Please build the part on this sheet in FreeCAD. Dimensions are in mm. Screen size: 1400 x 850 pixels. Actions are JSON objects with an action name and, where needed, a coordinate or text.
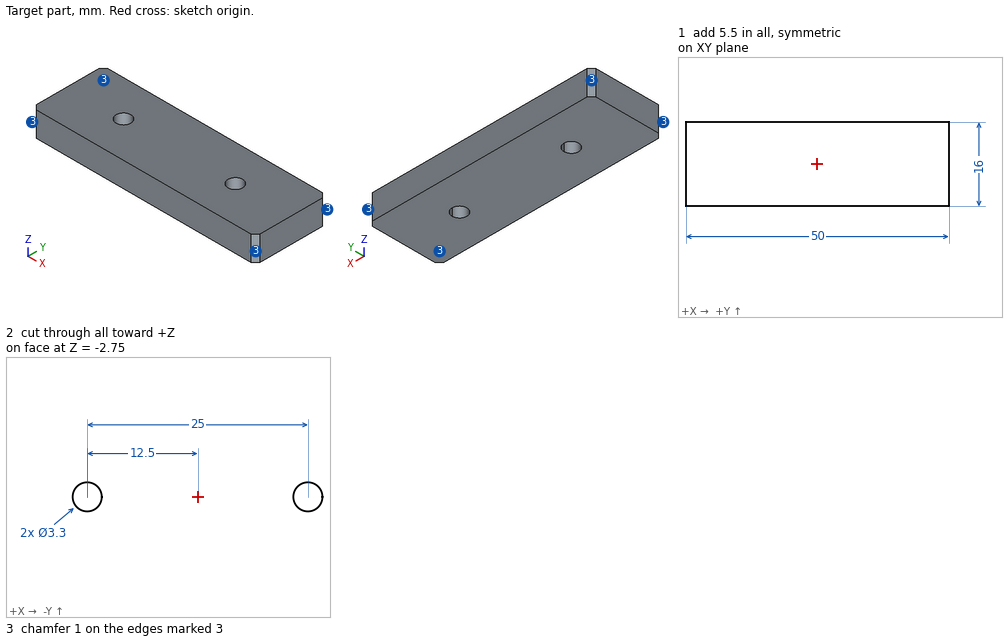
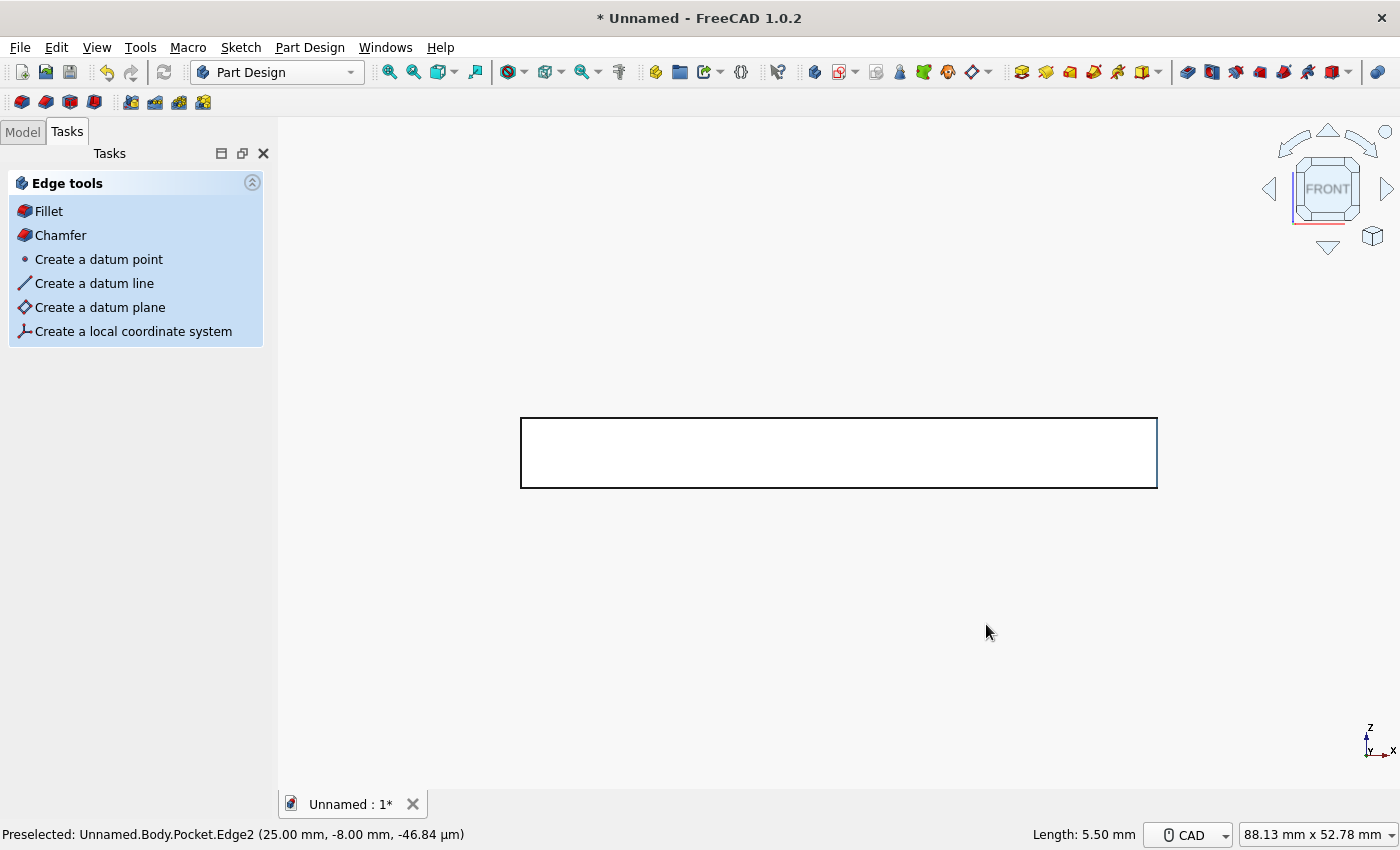
{"action": "left_click", "coordinate": [521, 452], "text": "ctrl"}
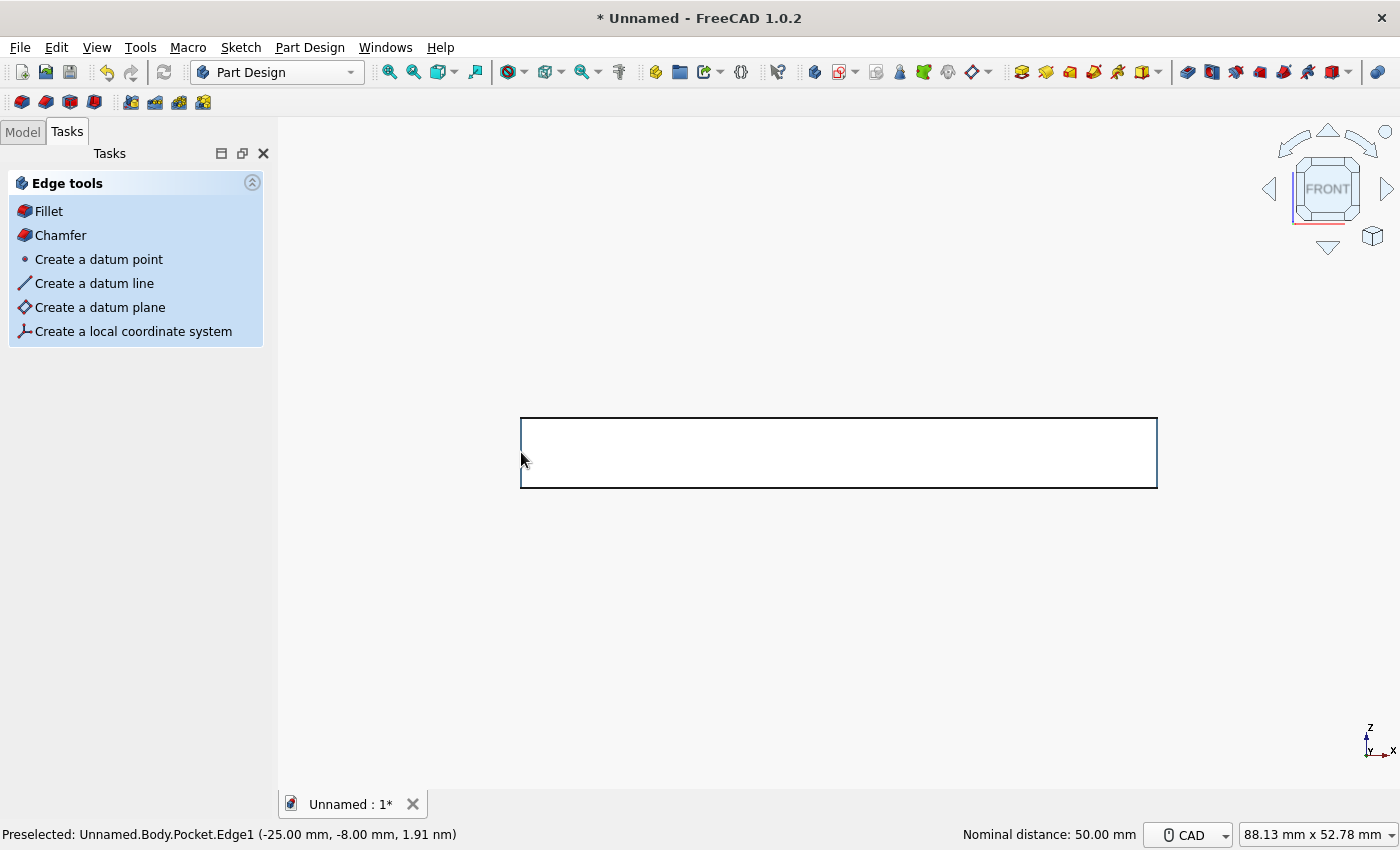
{"action": "key", "text": "3"}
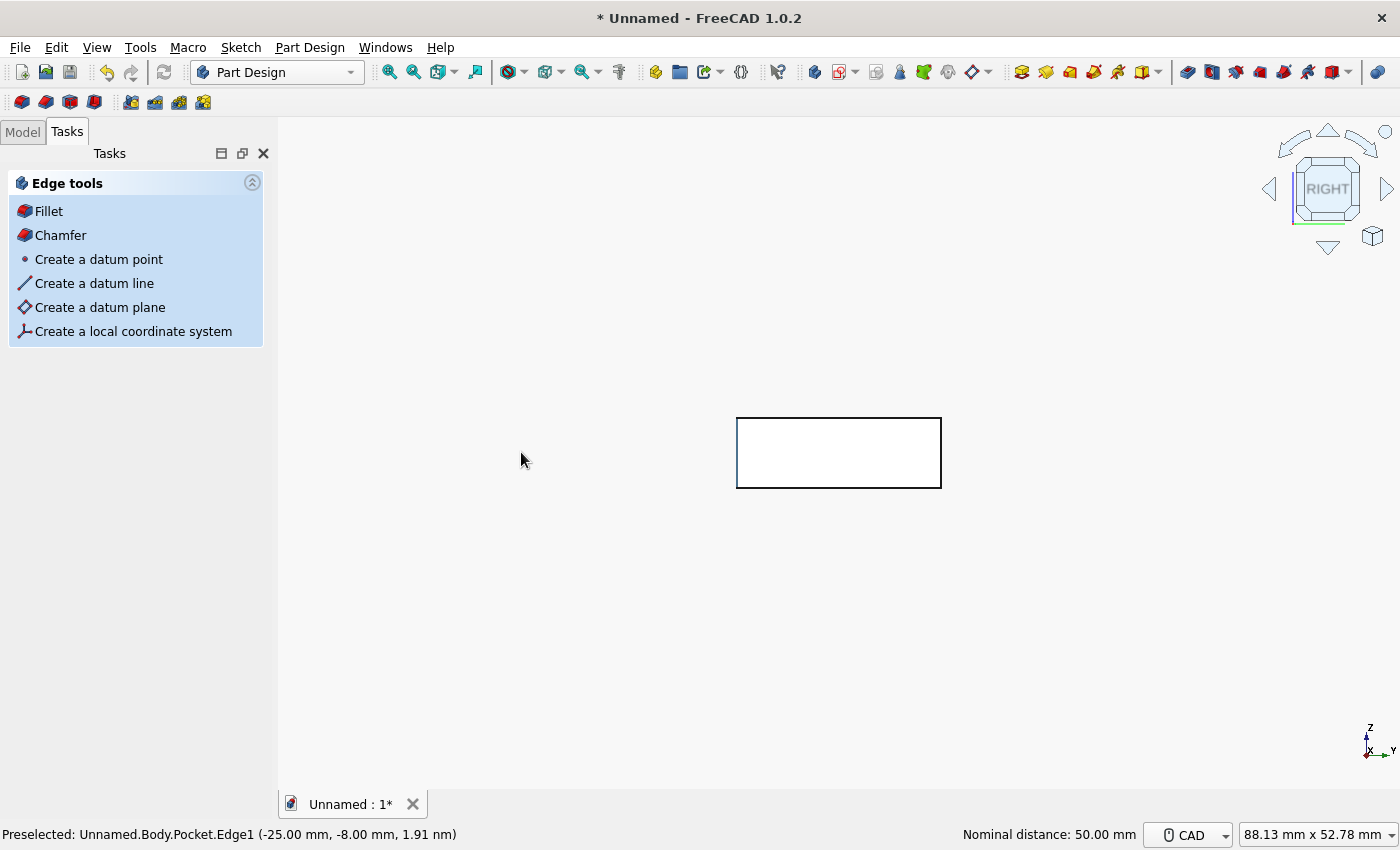
{"action": "key", "text": "v f"}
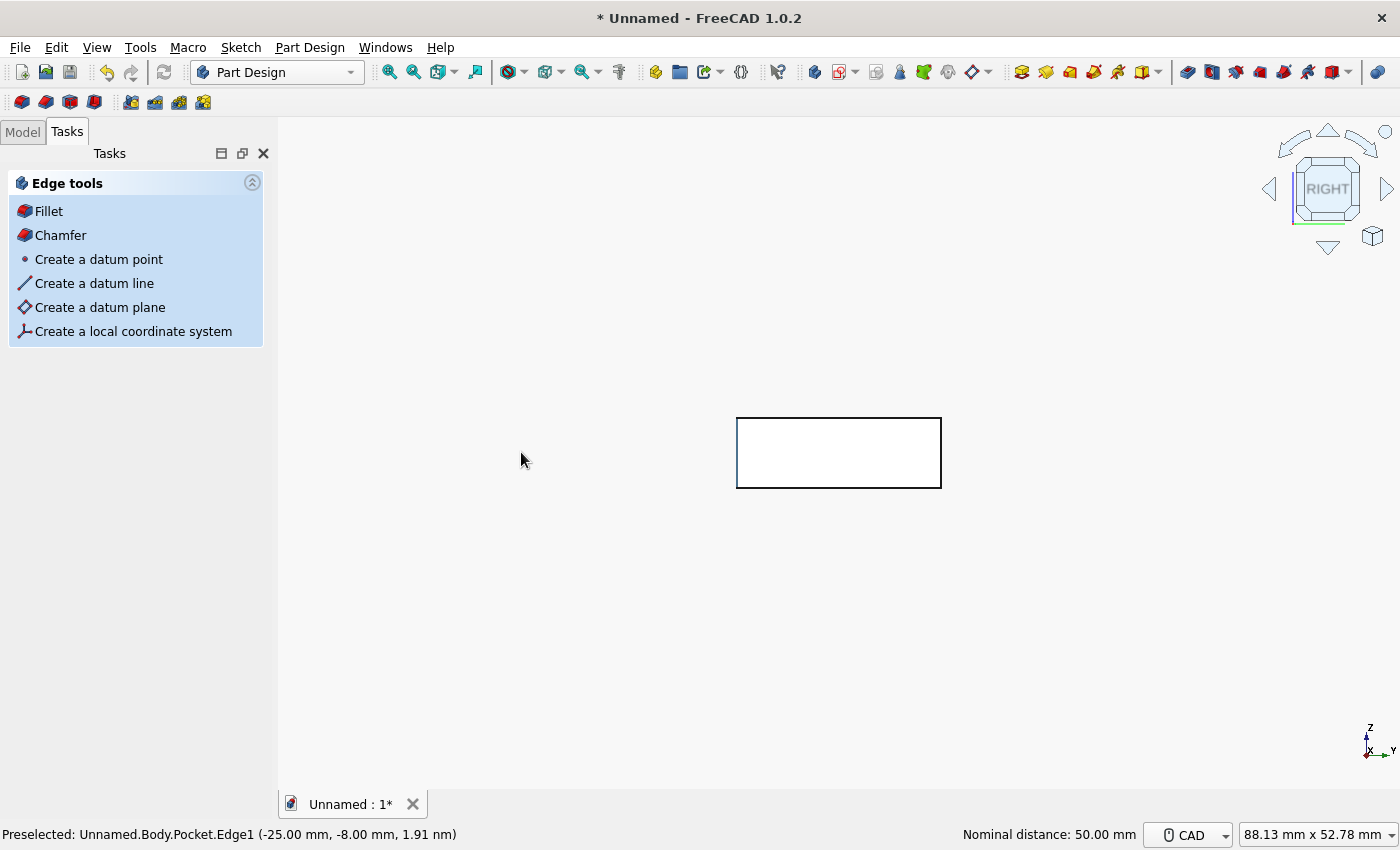
{"action": "left_click", "coordinate": [941, 452], "text": "ctrl"}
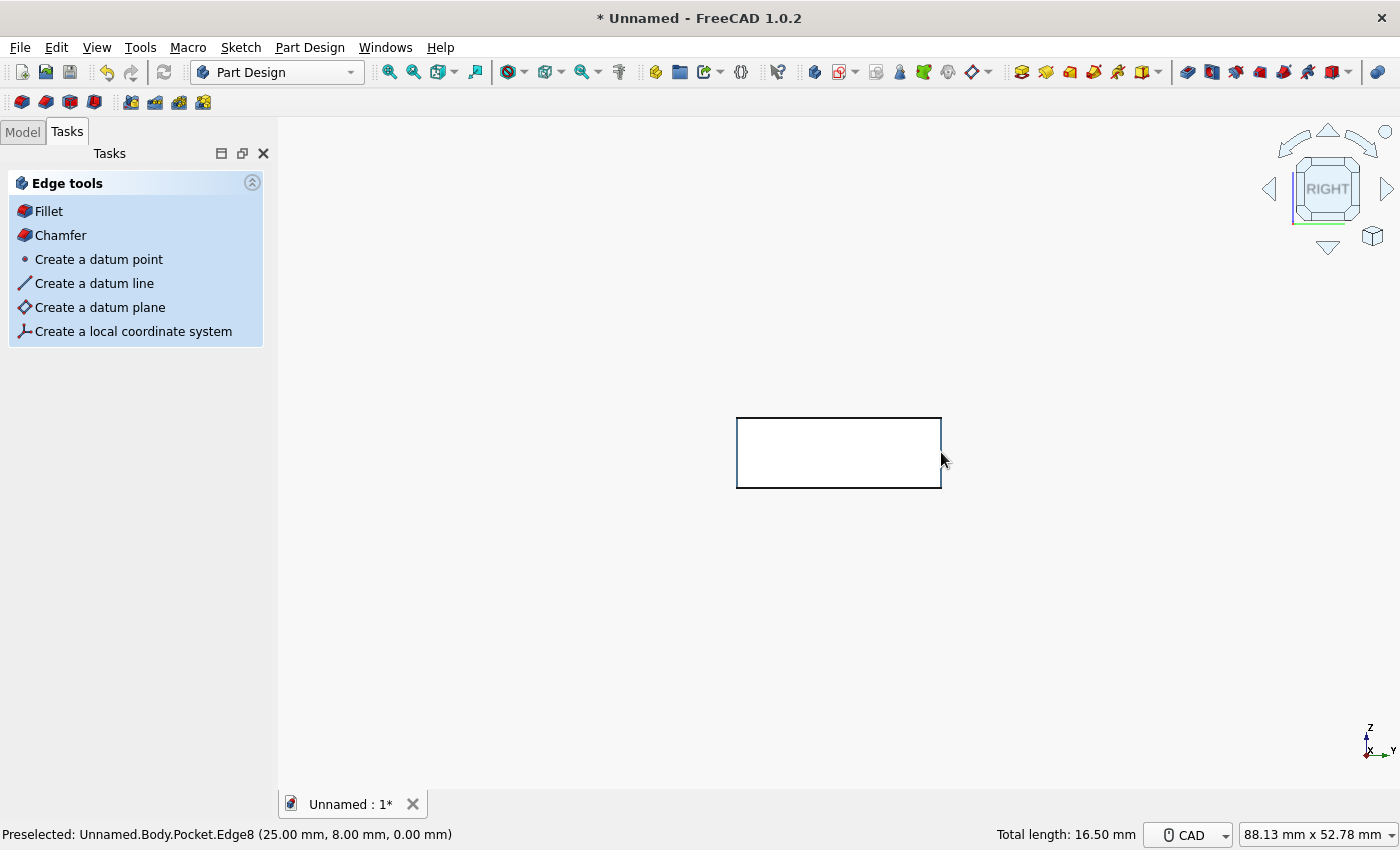
{"action": "key", "text": "5"}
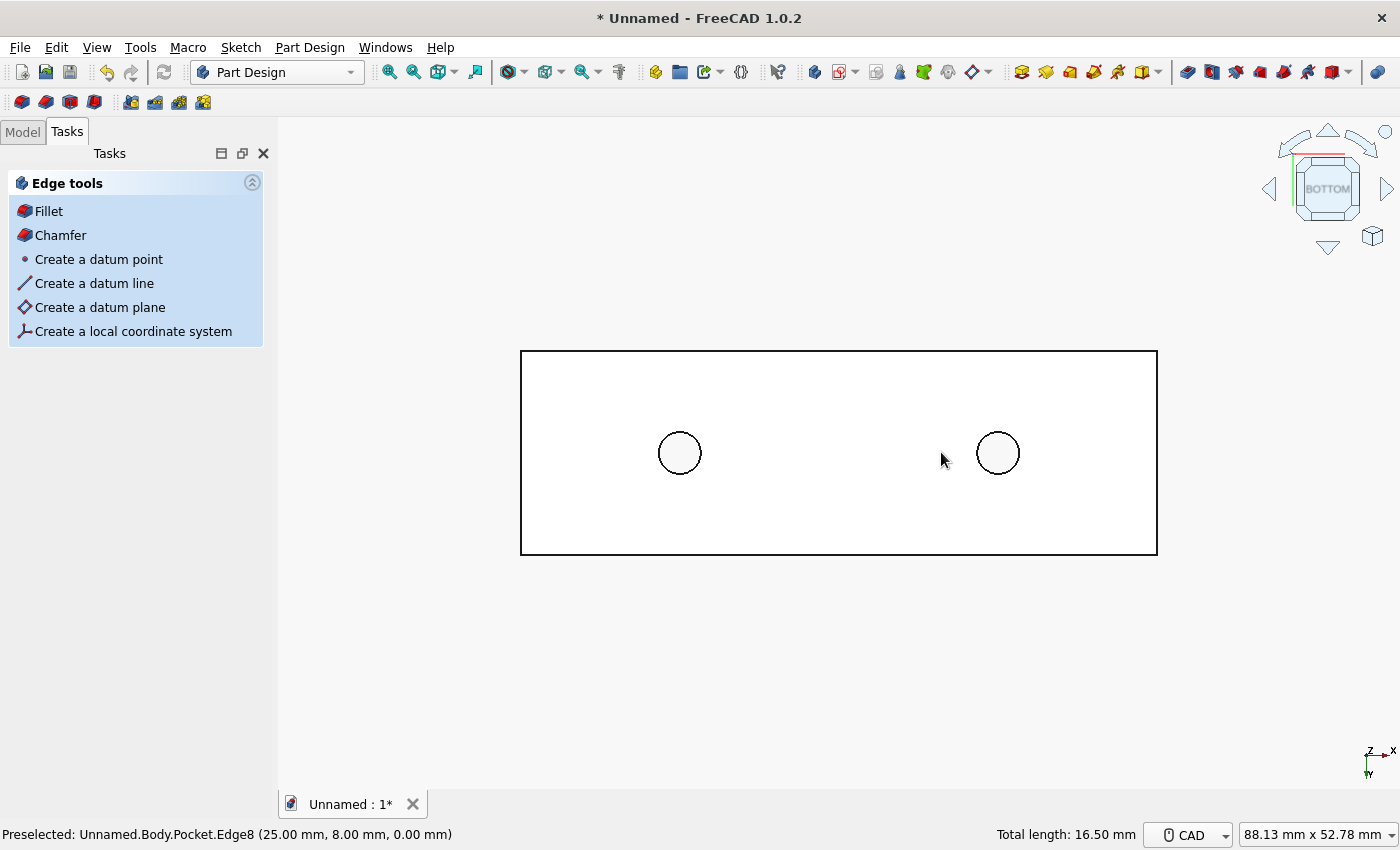
{"action": "key", "text": "4"}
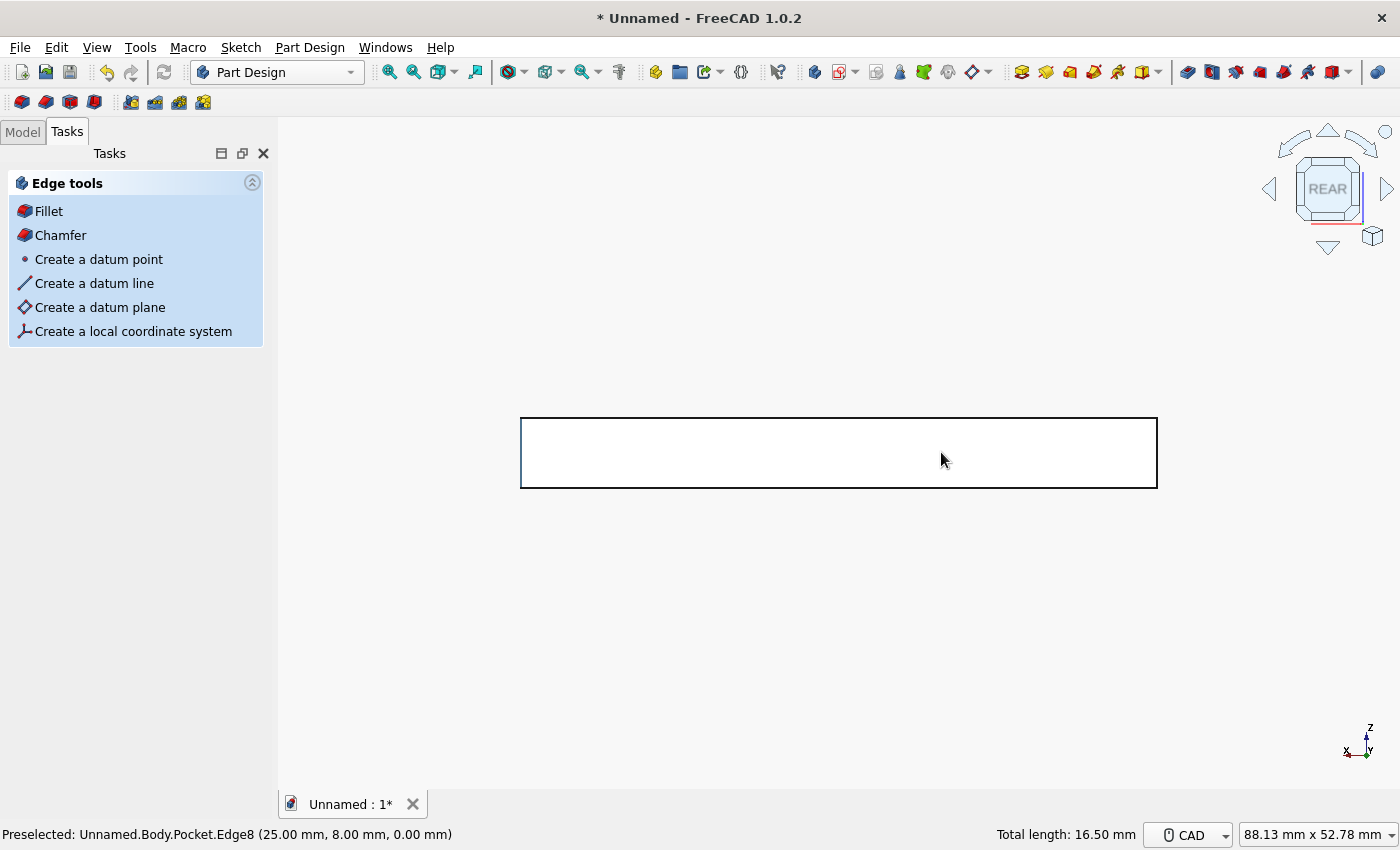
{"action": "left_click", "coordinate": [1157, 452], "text": "ctrl"}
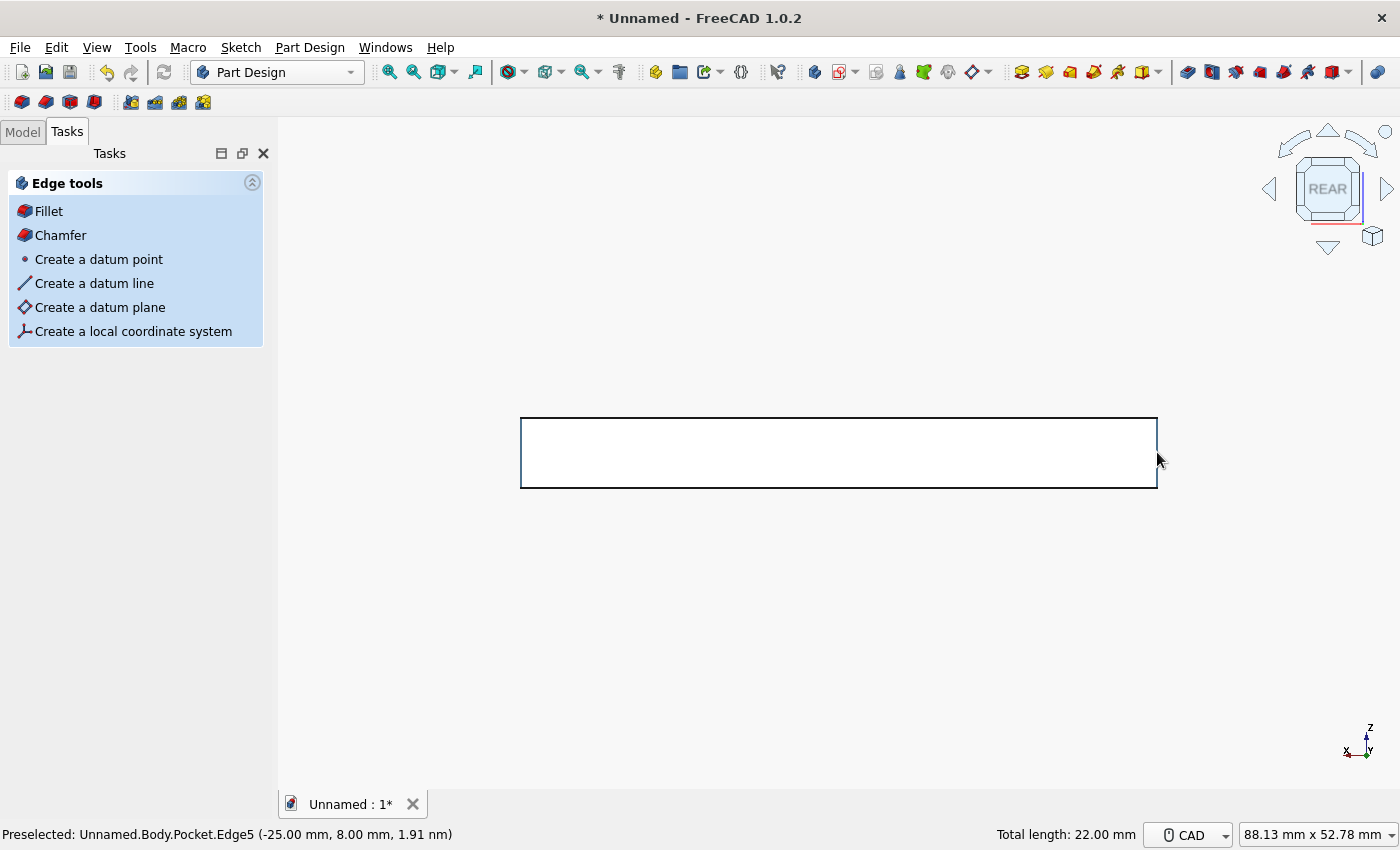
{"action": "left_click", "coordinate": [46, 102]}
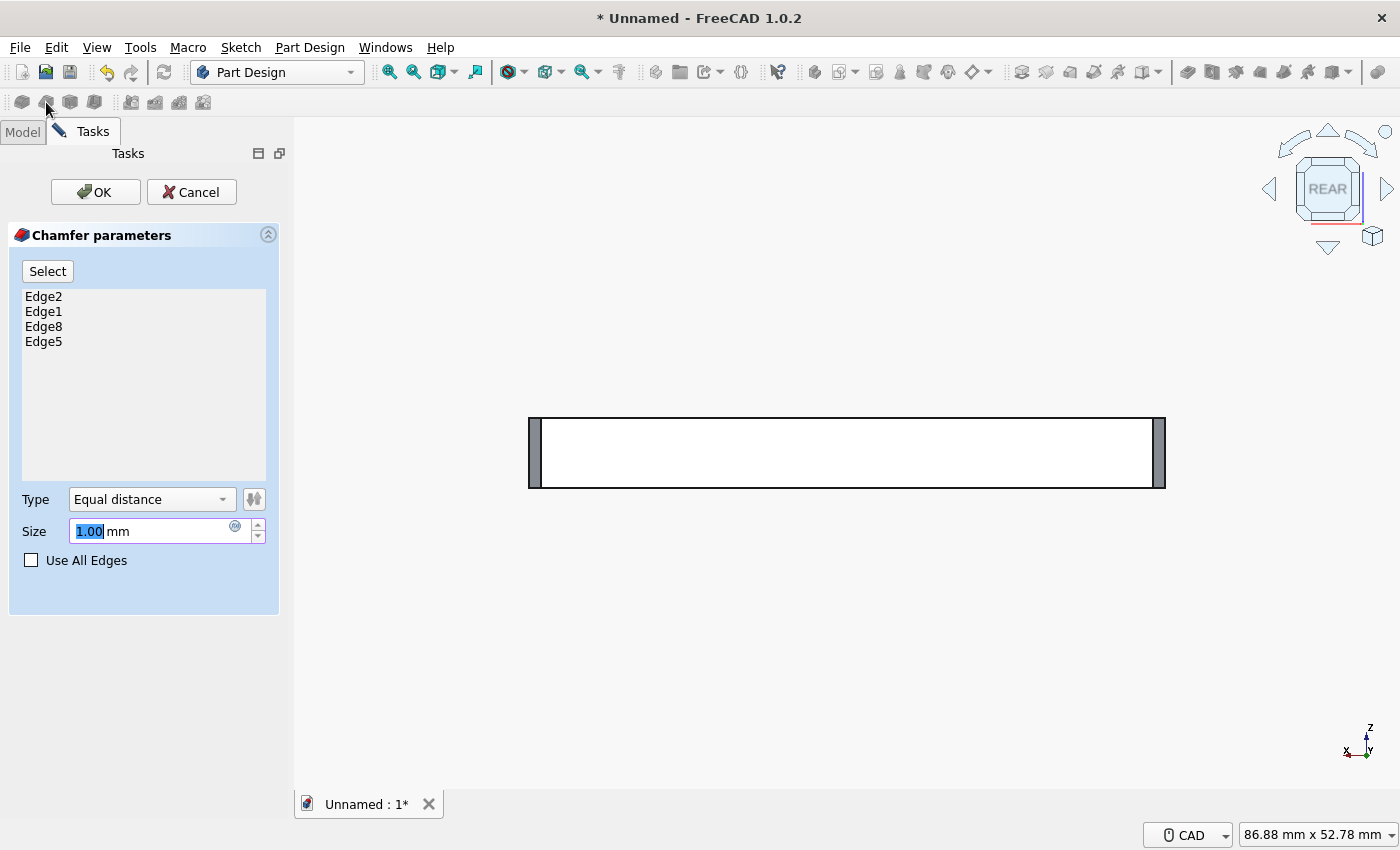
{"action": "type", "text": "1"}
{"action": "key", "text": "Tab"}